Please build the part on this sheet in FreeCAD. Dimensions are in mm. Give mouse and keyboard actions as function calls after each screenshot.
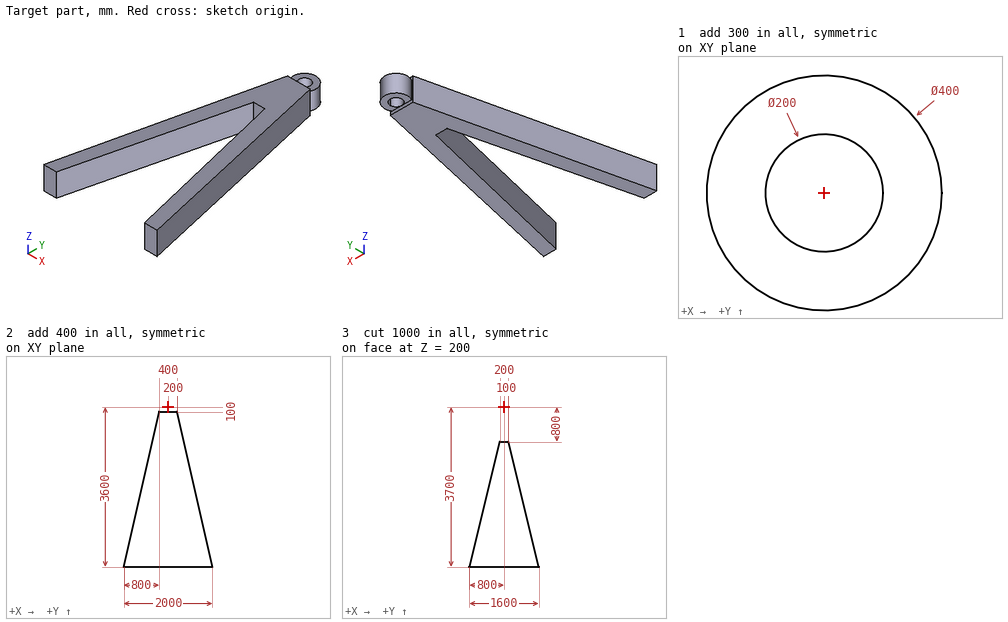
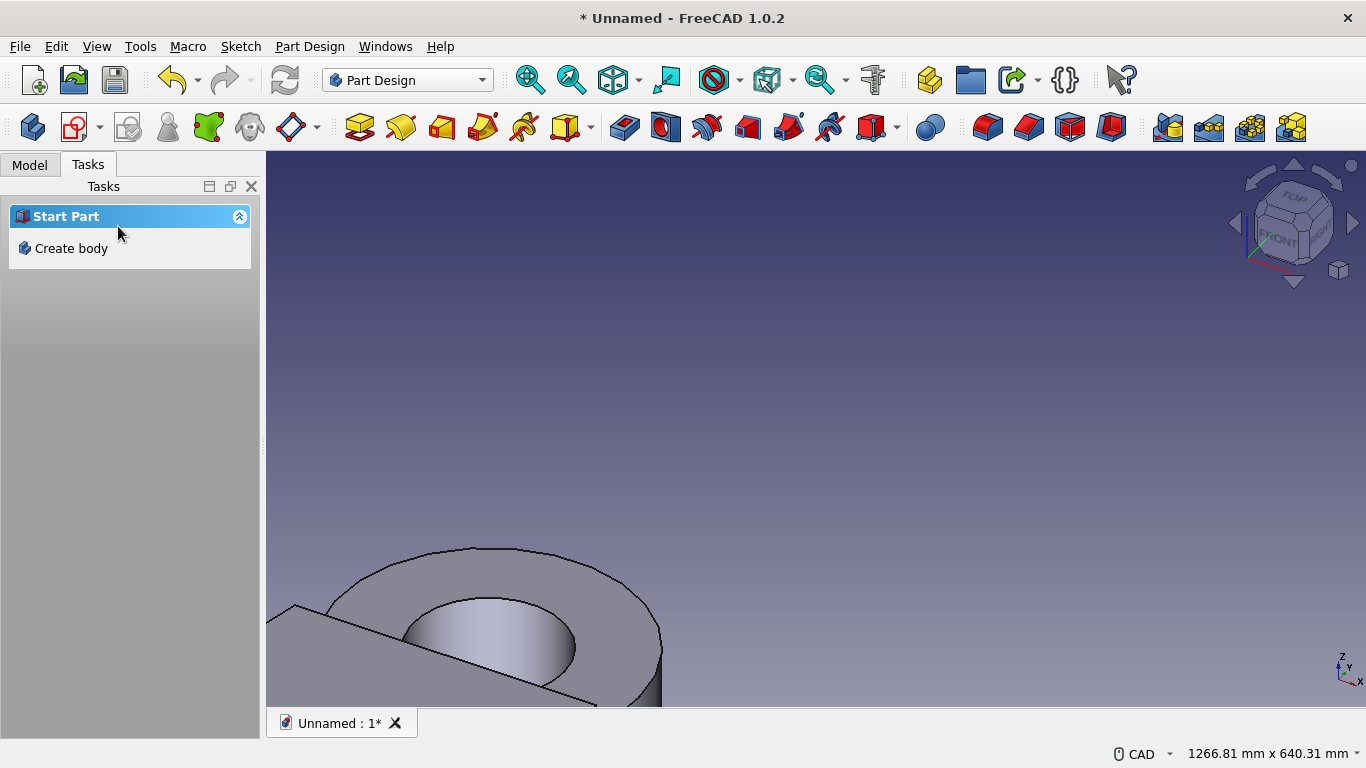
click(531, 80)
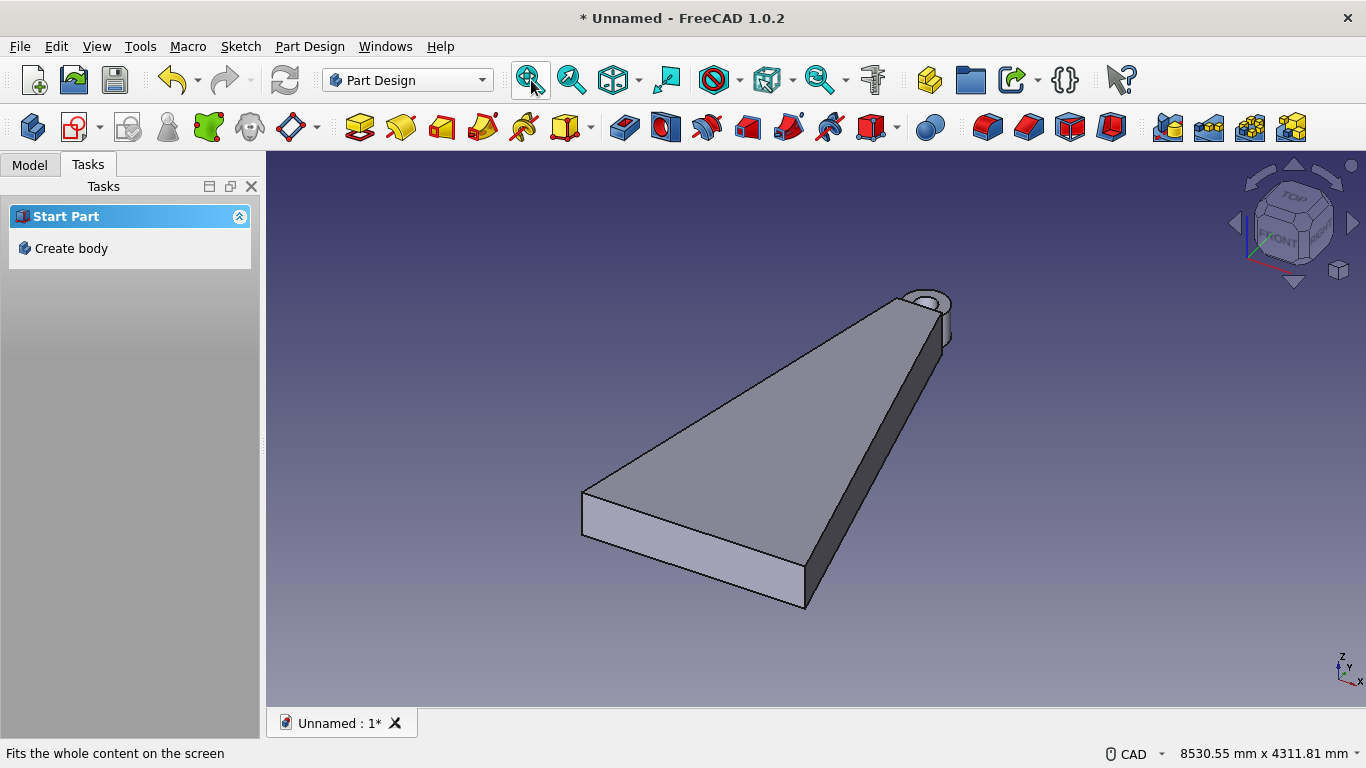
click(742, 480)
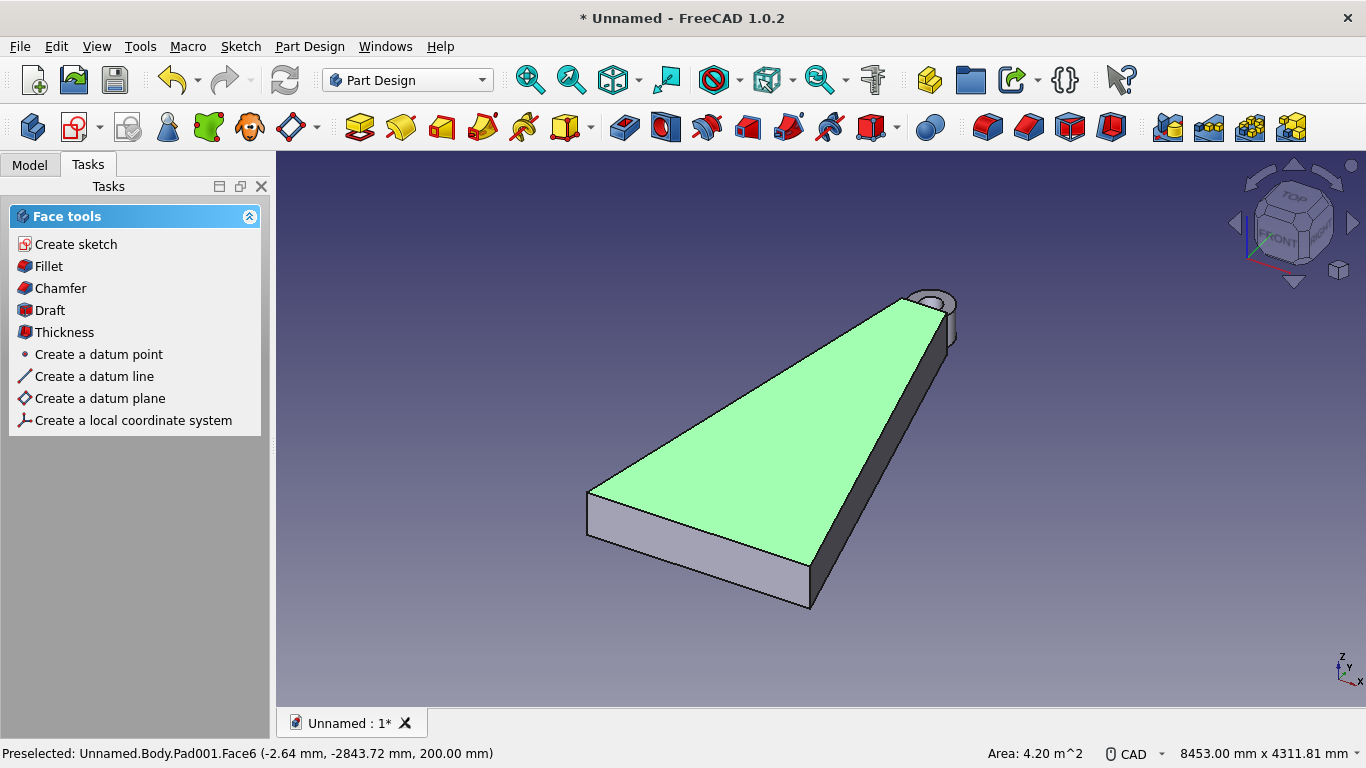
click(74, 128)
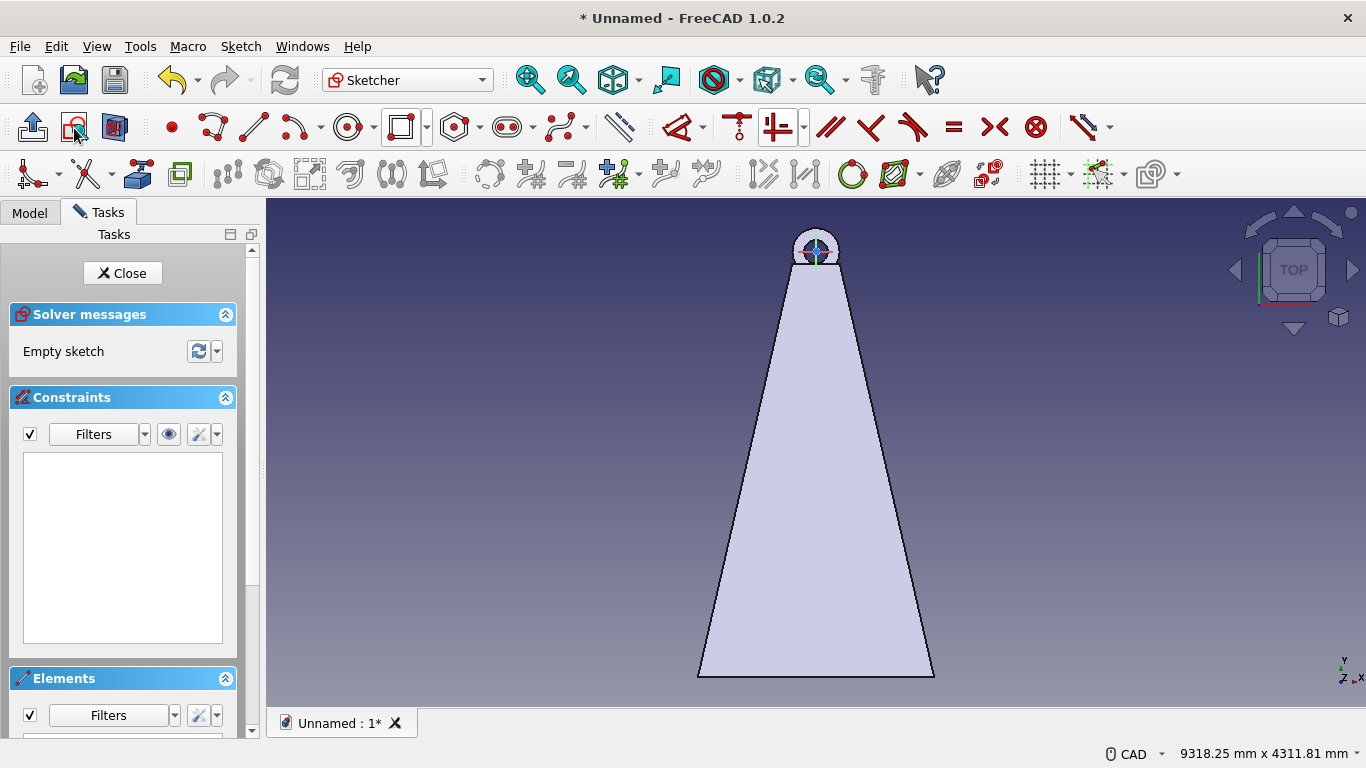
scroll(608, 417, down, 2)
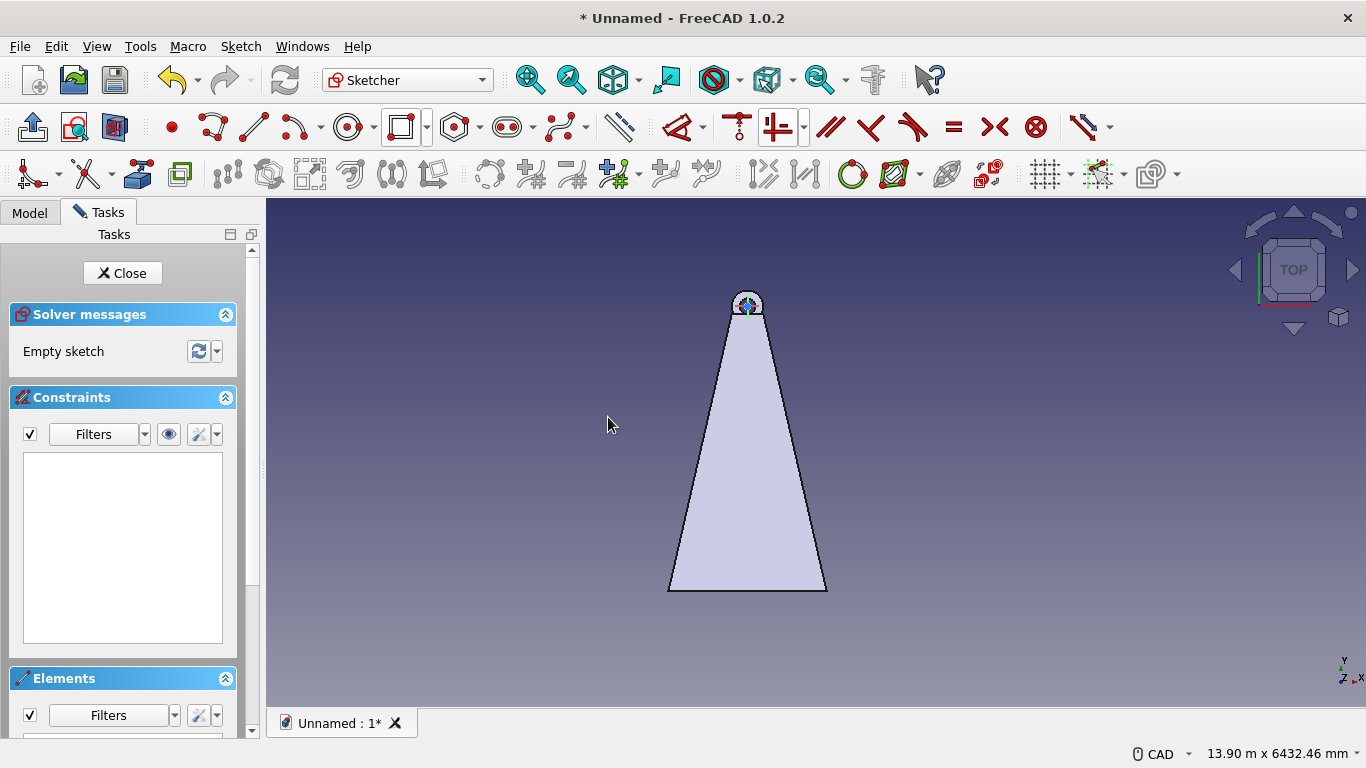
click(213, 128)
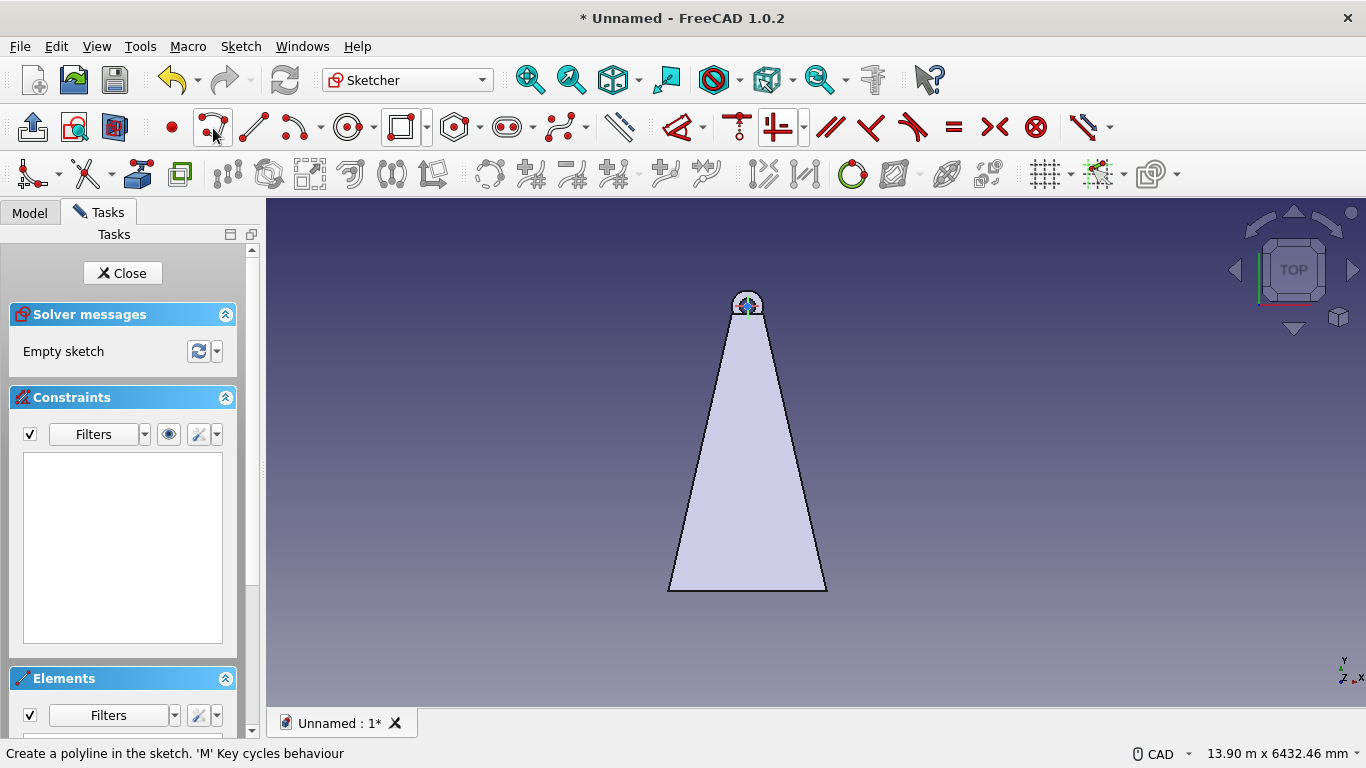
scroll(755, 370, up, 4)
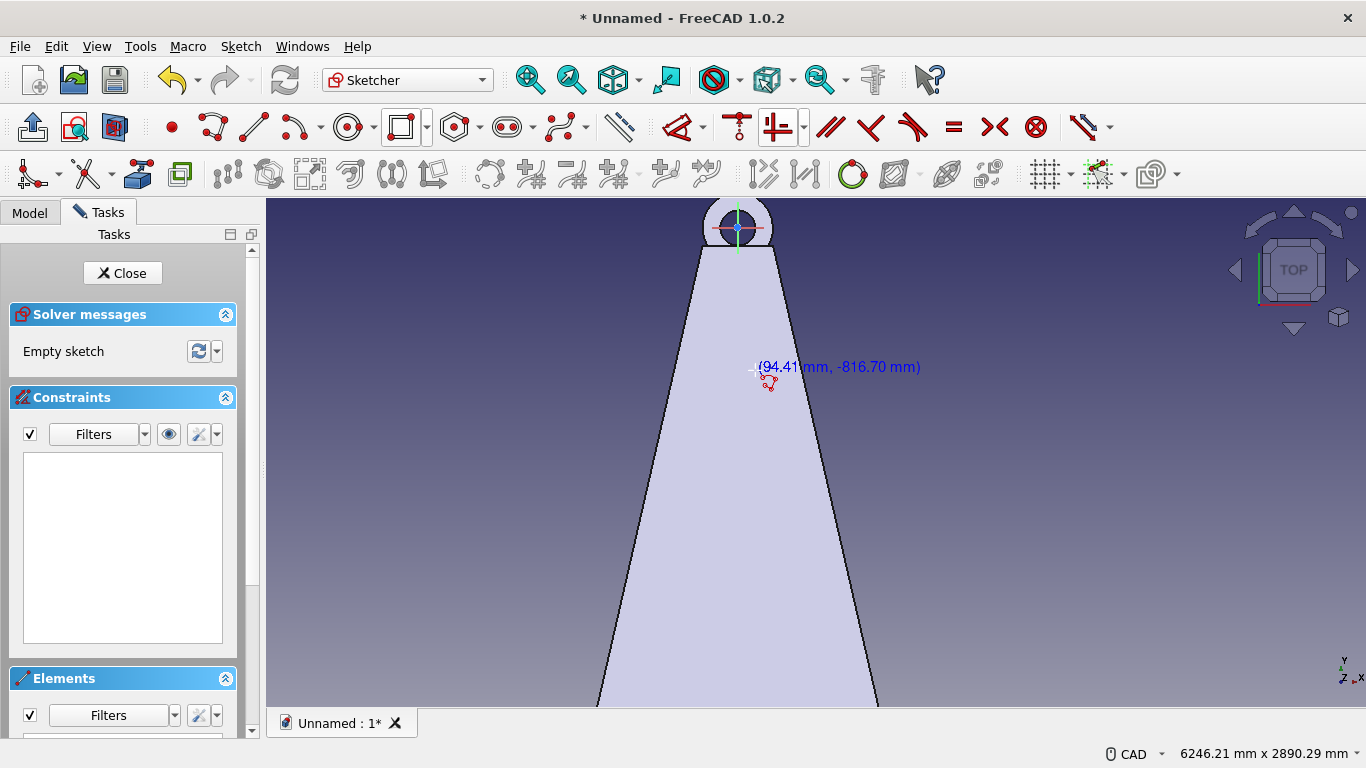
click(755, 369)
click(720, 369)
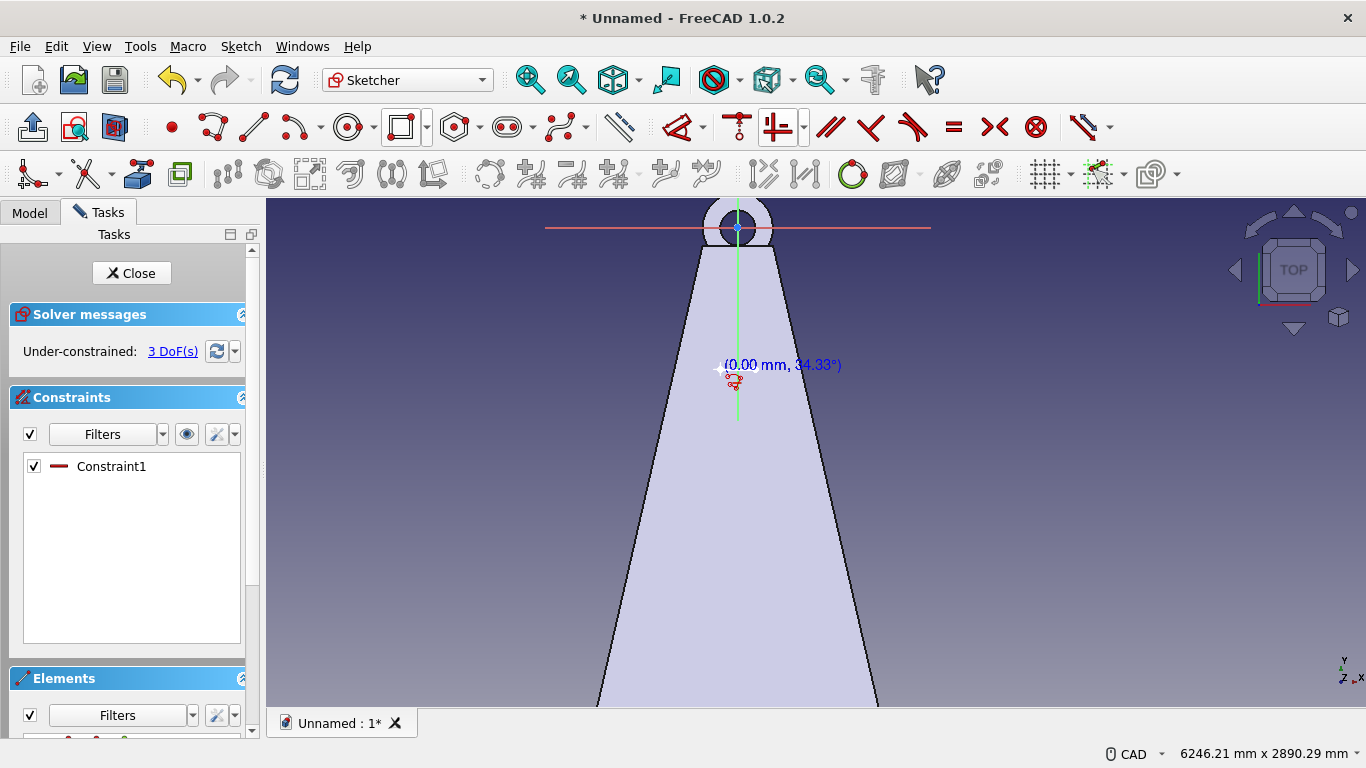
scroll(755, 370, down, 4)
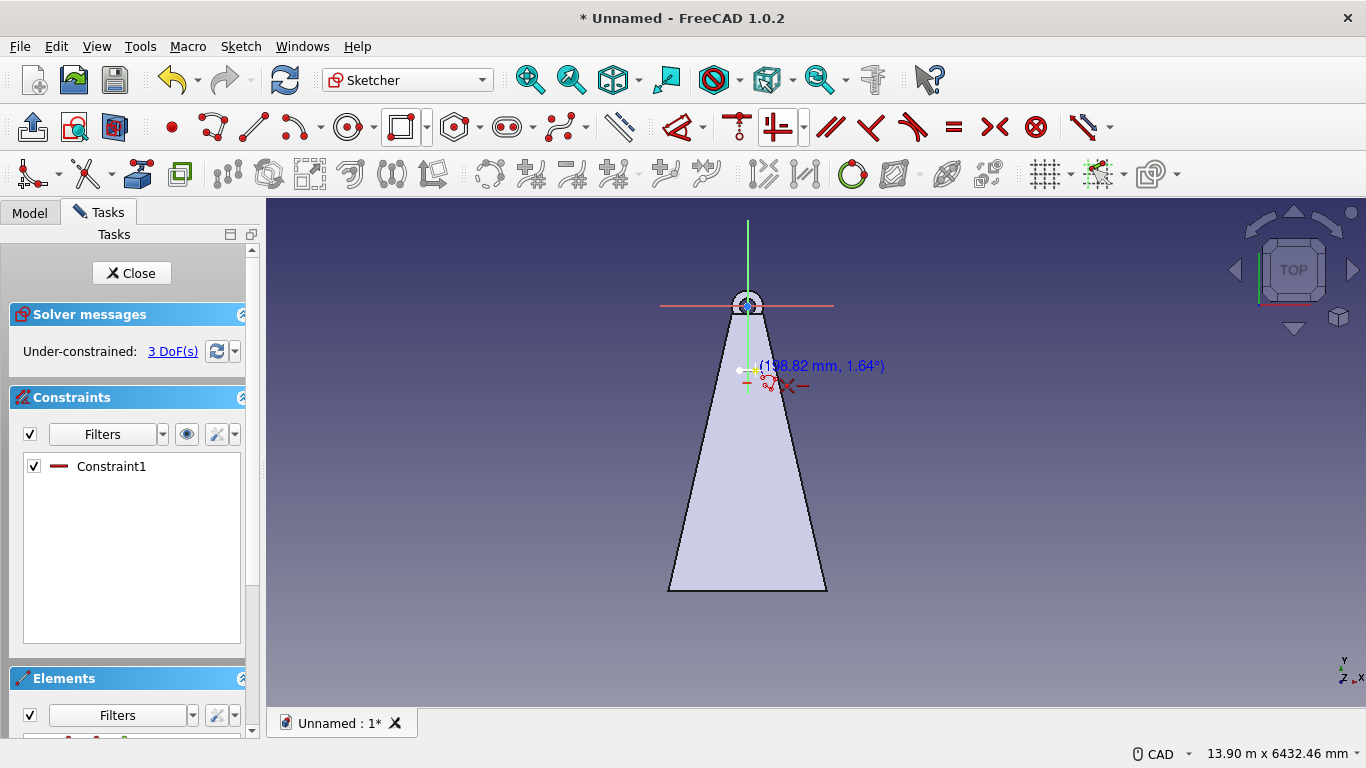
click(684, 599)
click(811, 599)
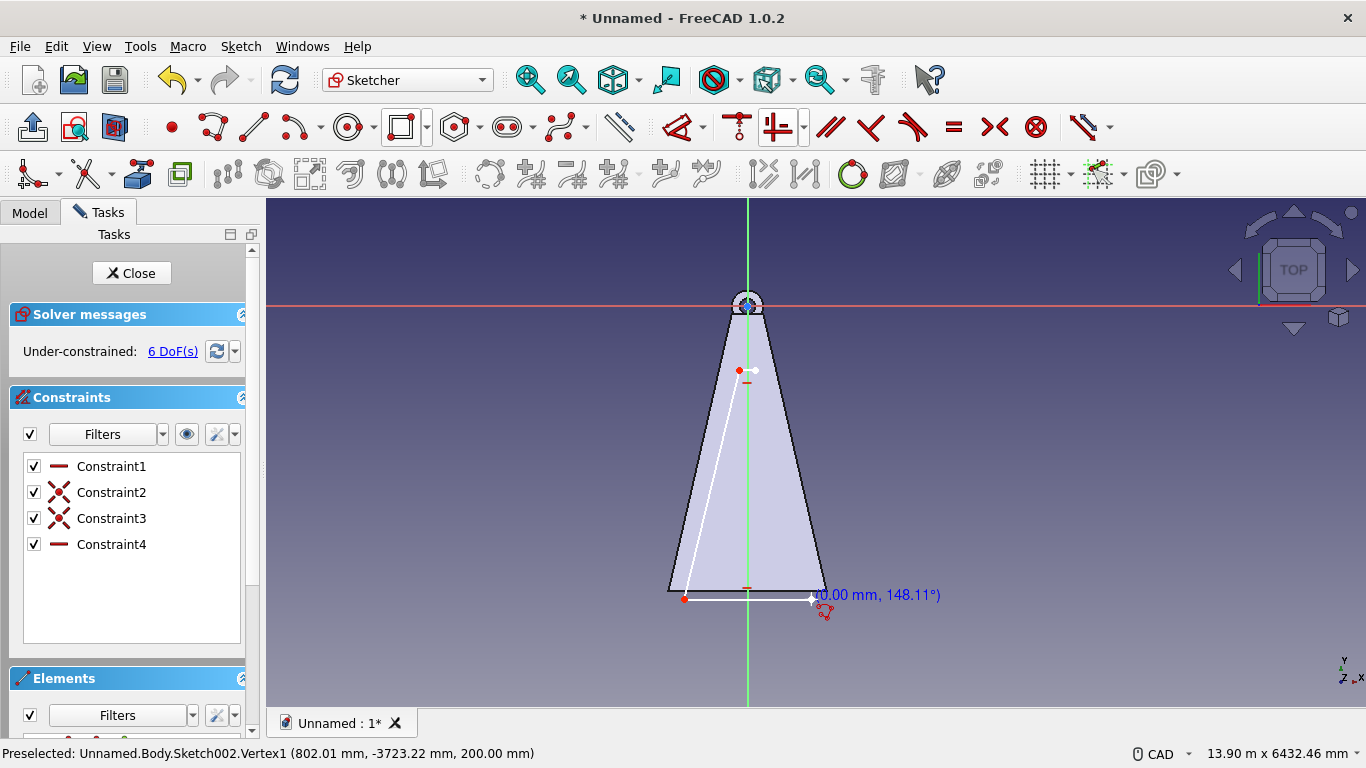
scroll(755, 370, up, 4)